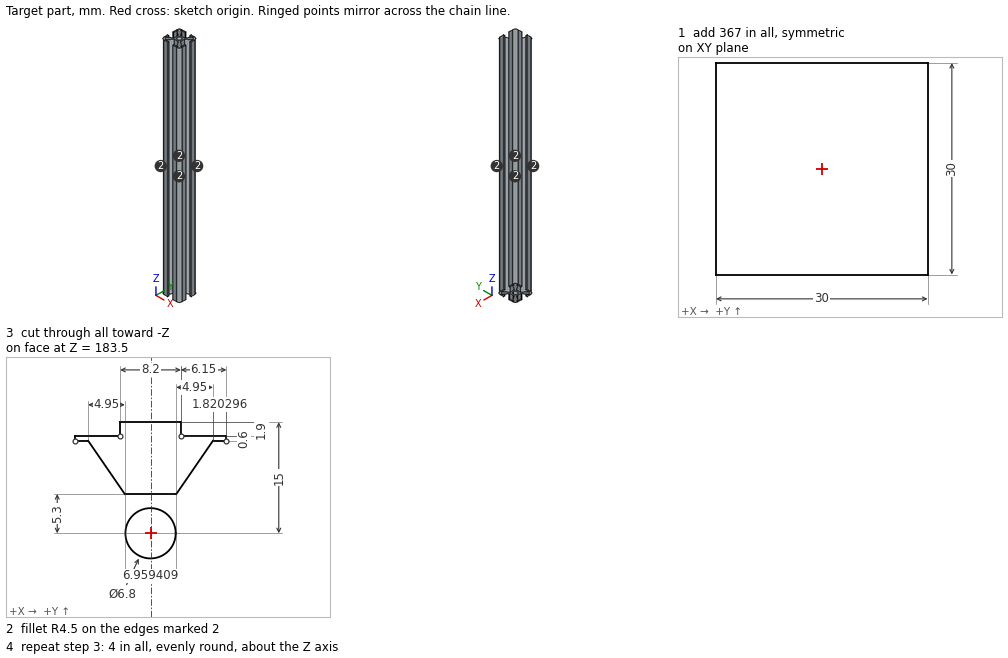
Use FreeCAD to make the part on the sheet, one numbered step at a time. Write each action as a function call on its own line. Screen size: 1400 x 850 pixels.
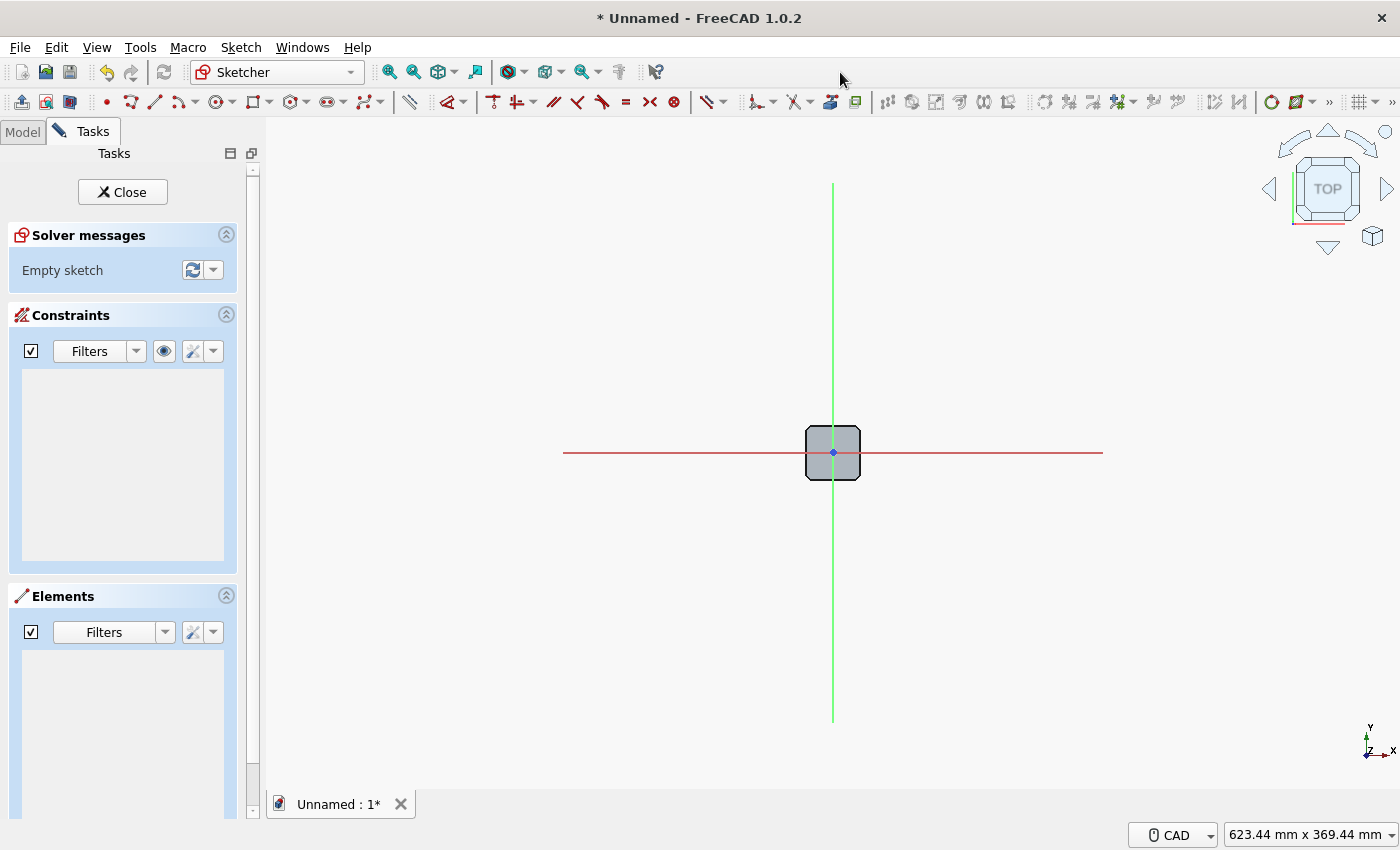
scroll(838, 442, up, 13)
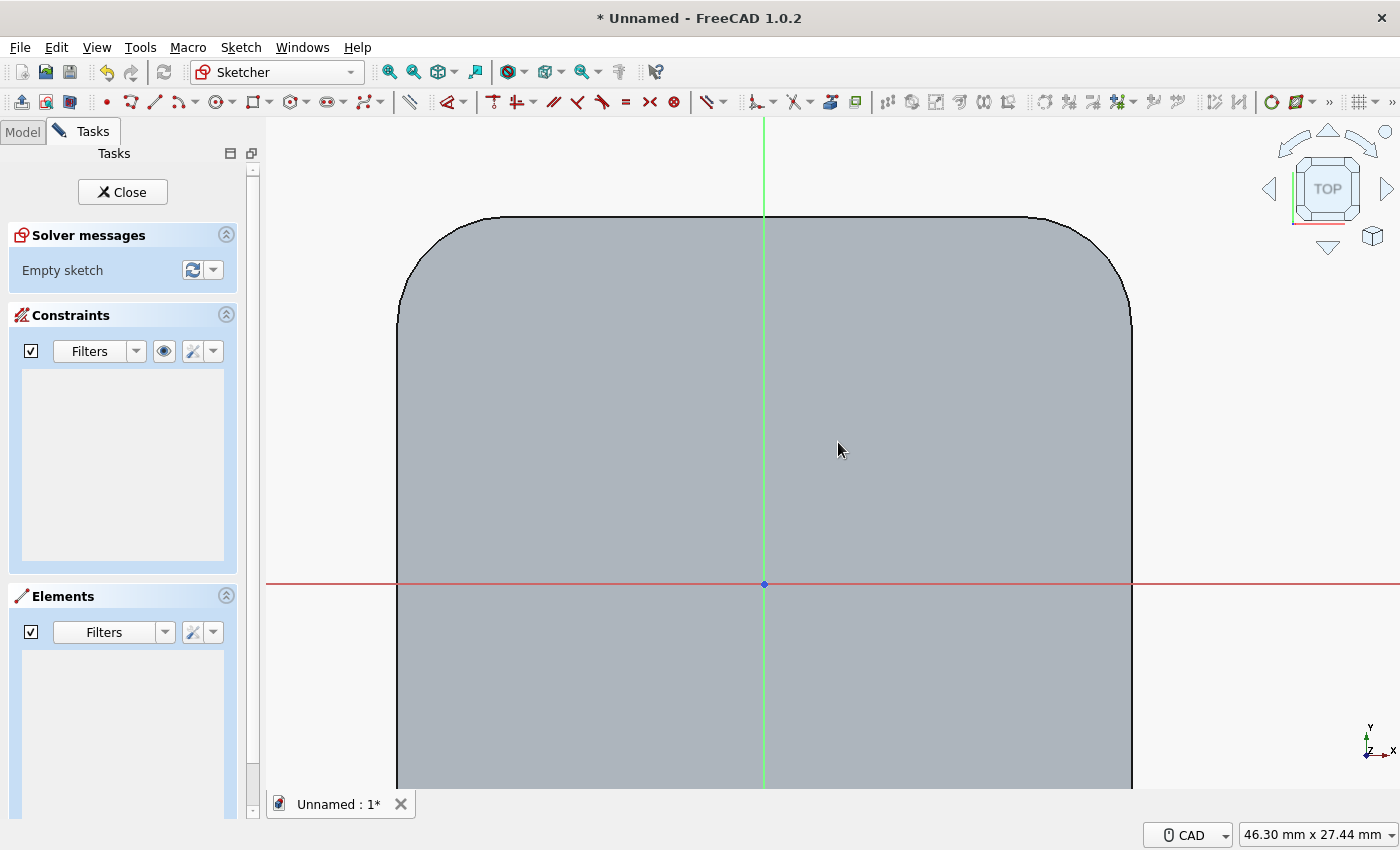
key(g)
key(m)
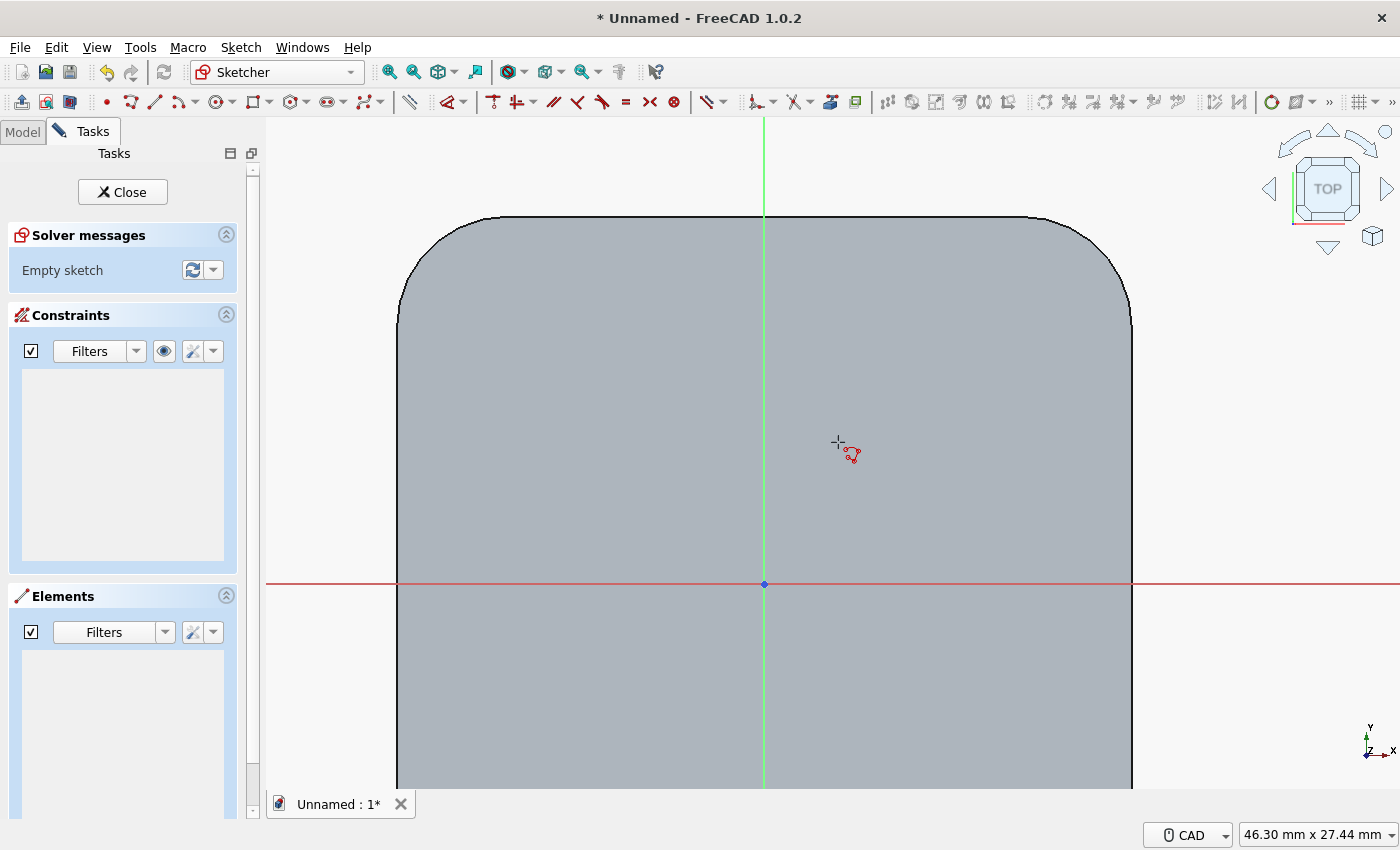
click(679, 454)
click(850, 454)
click(971, 278)
click(1015, 278)
click(1015, 263)
click(865, 263)
click(865, 217)
click(664, 217)
click(664, 263)
click(513, 263)
click(513, 278)
click(558, 278)
click(679, 455)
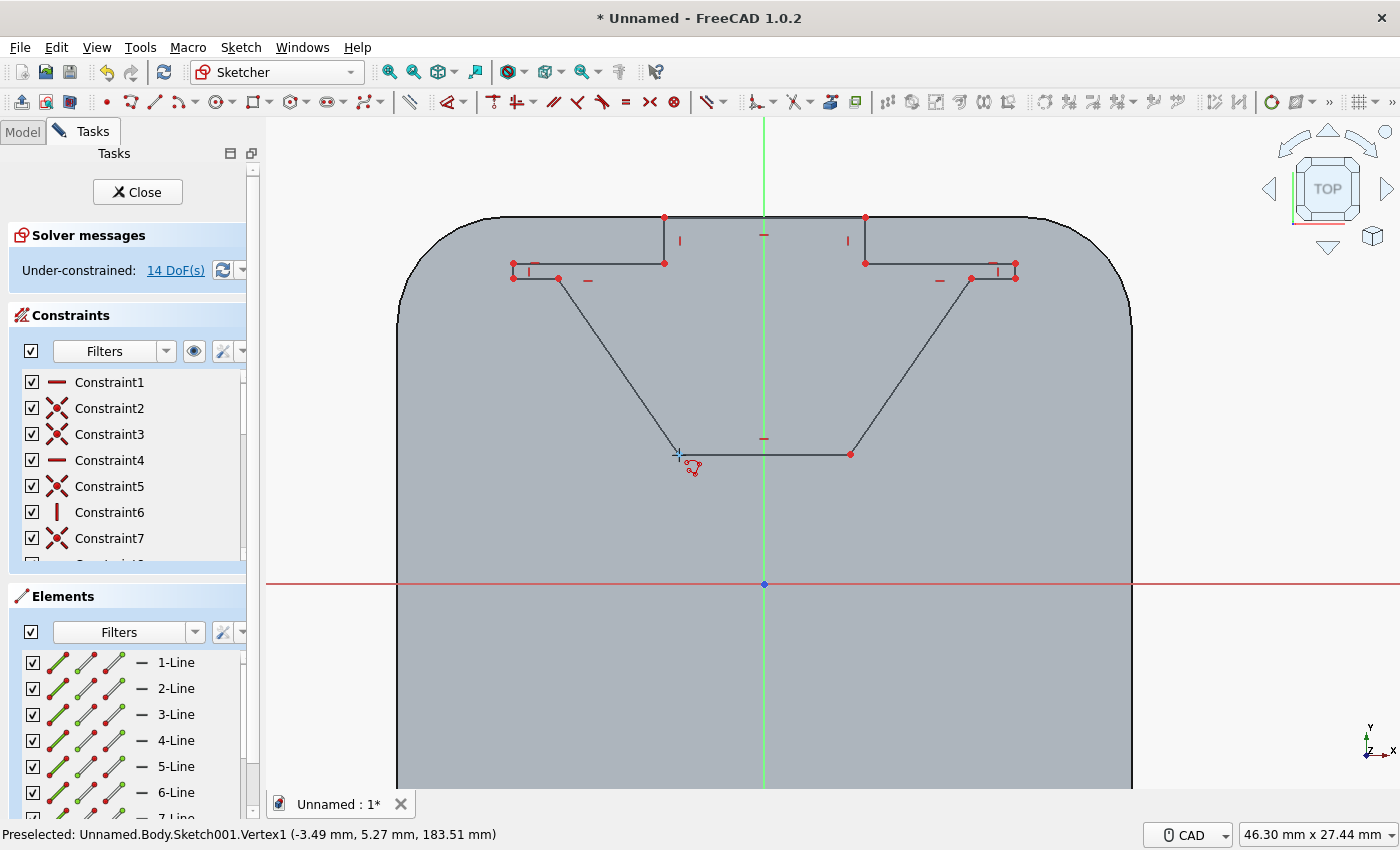
key(g)
key(c)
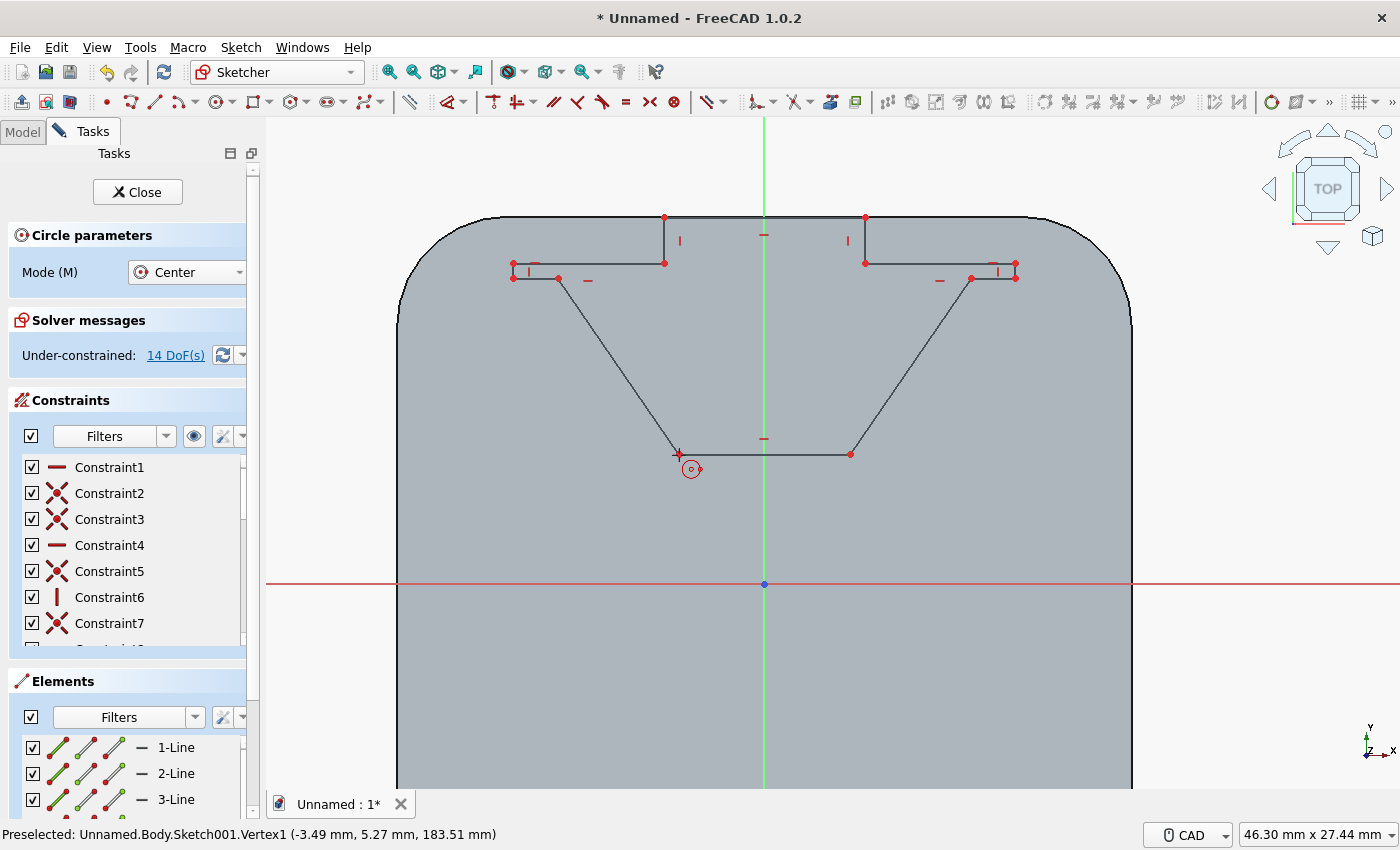
click(764, 584)
click(823, 525)
key(Escape)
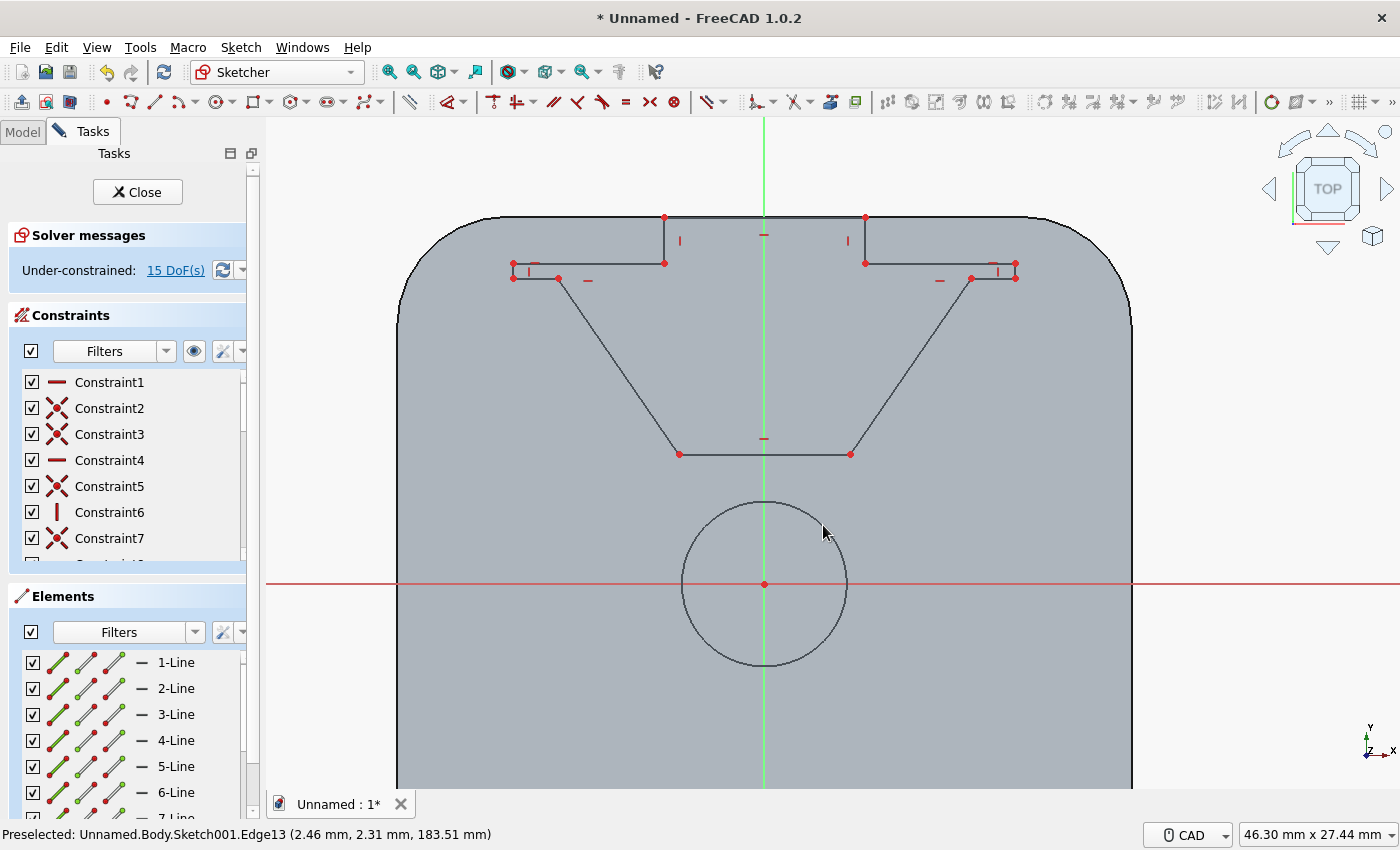
click(865, 264)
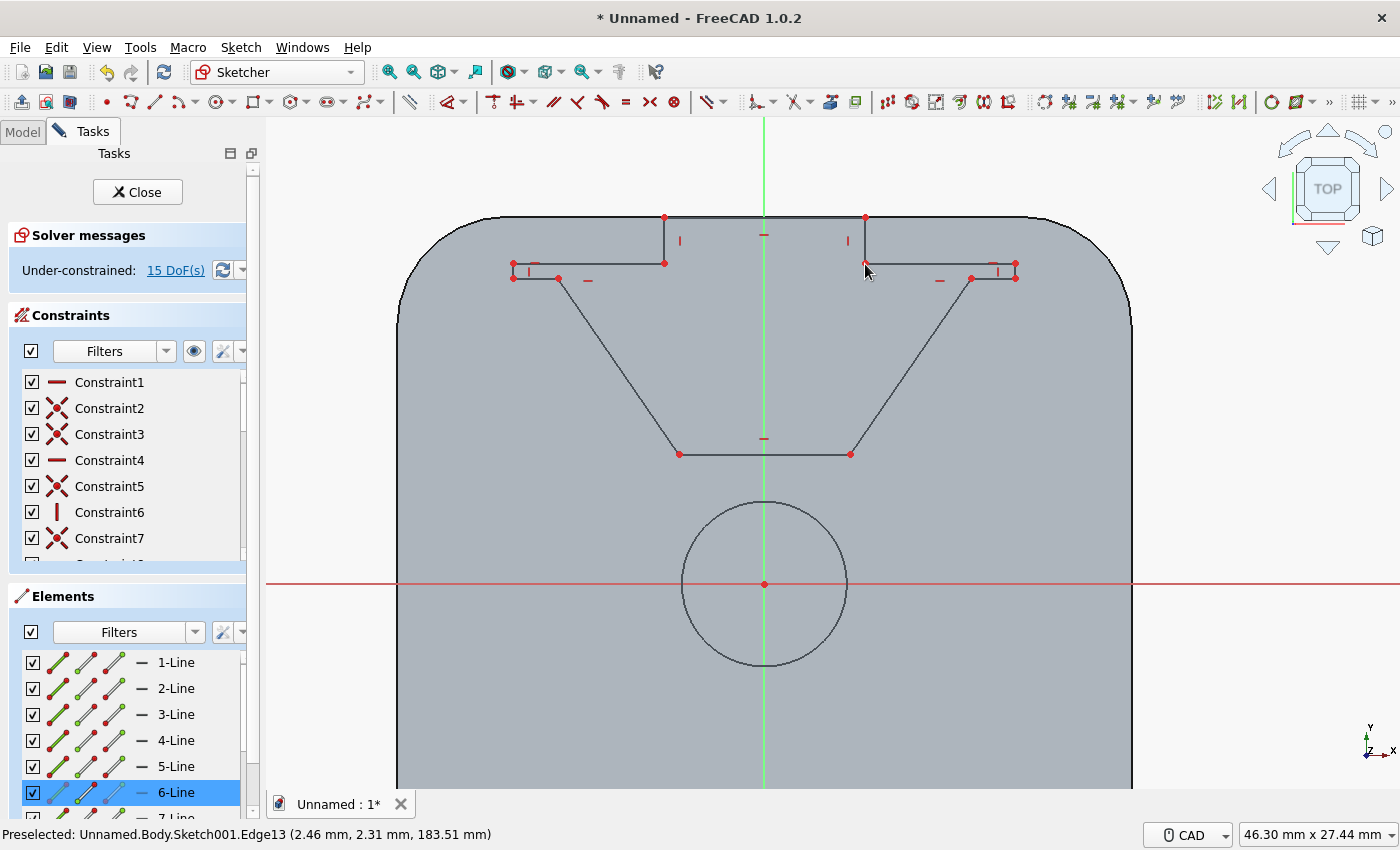
click(664, 264)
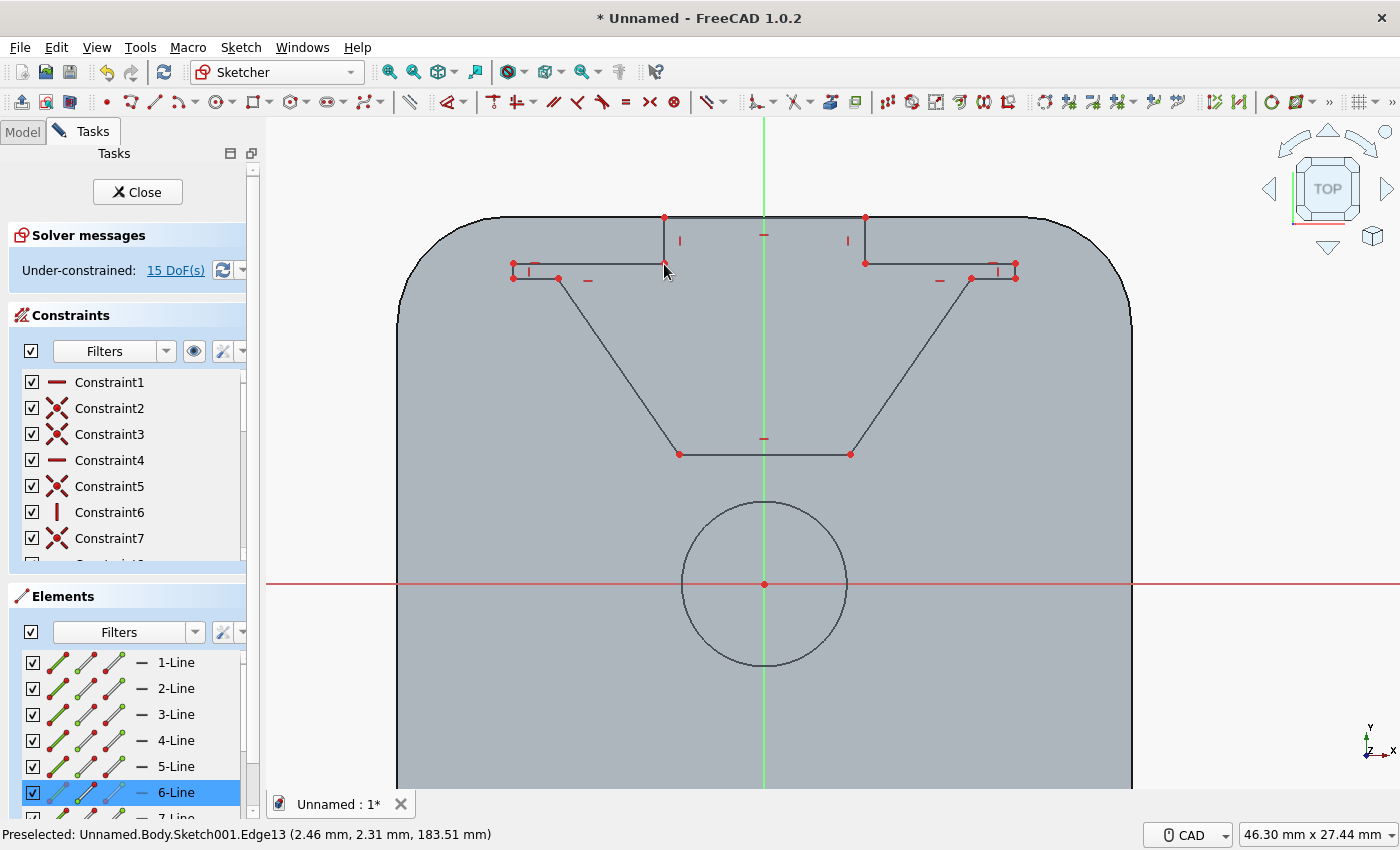
click(764, 717)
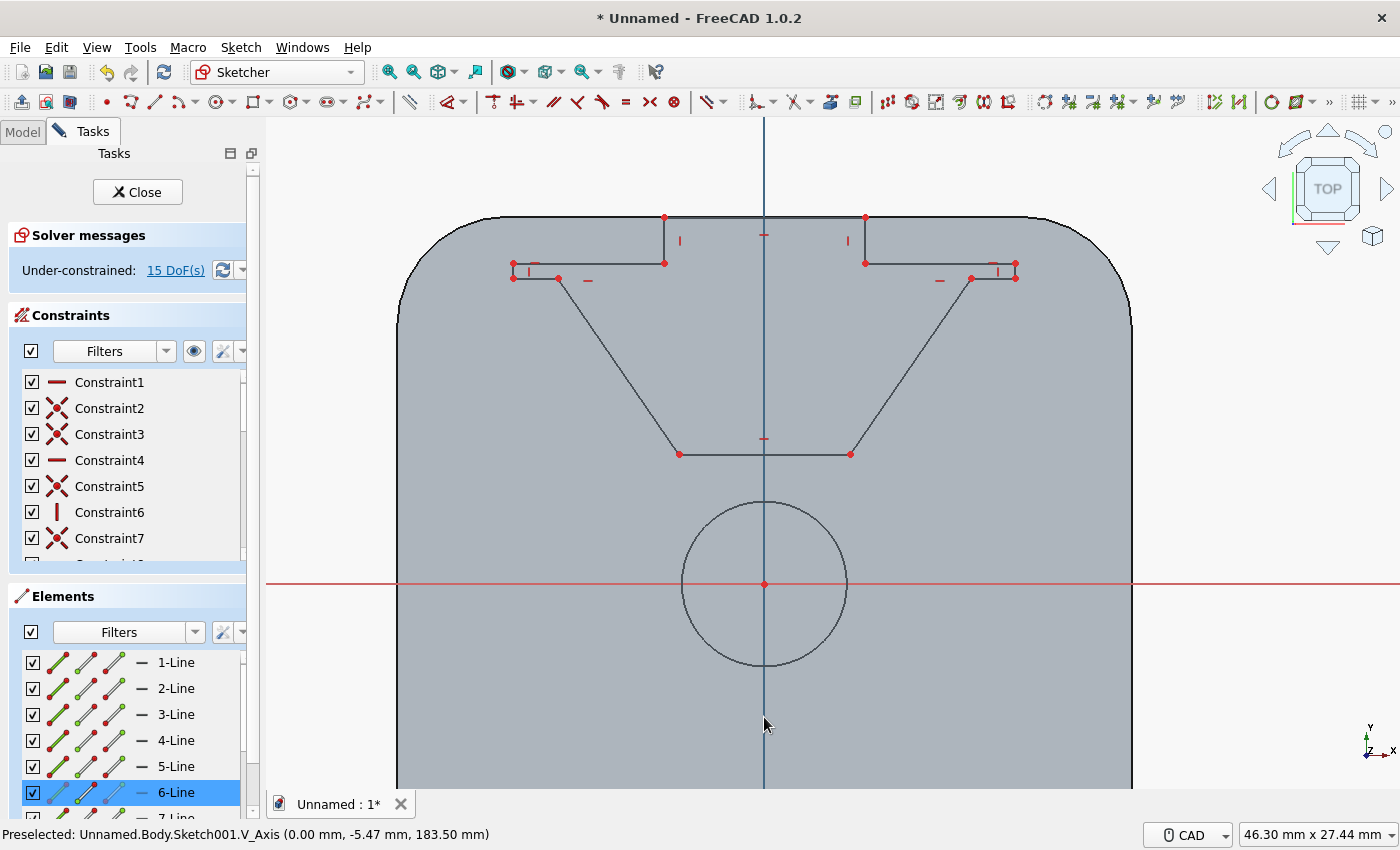
key(s)